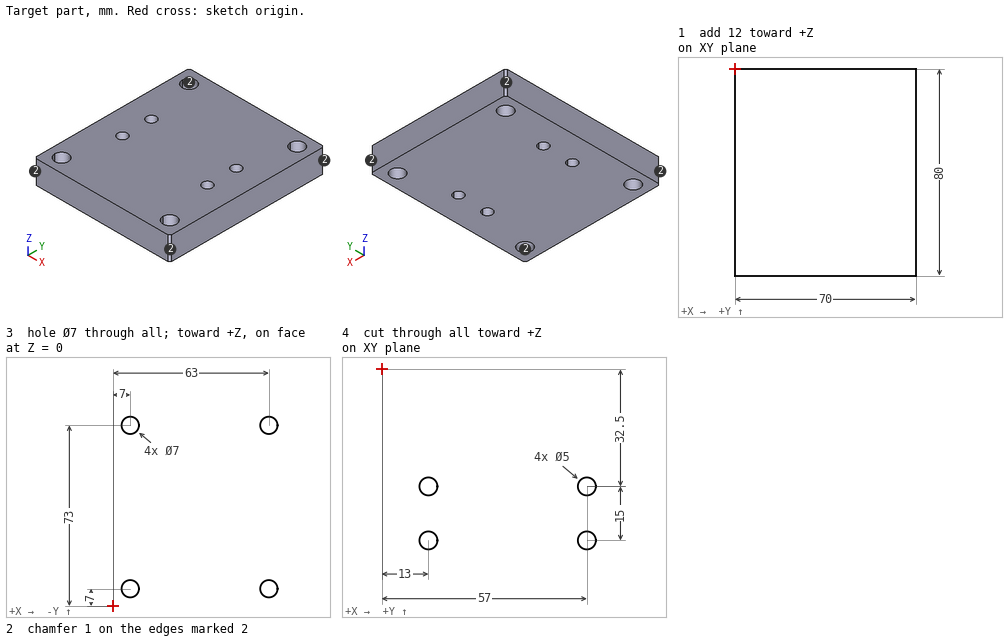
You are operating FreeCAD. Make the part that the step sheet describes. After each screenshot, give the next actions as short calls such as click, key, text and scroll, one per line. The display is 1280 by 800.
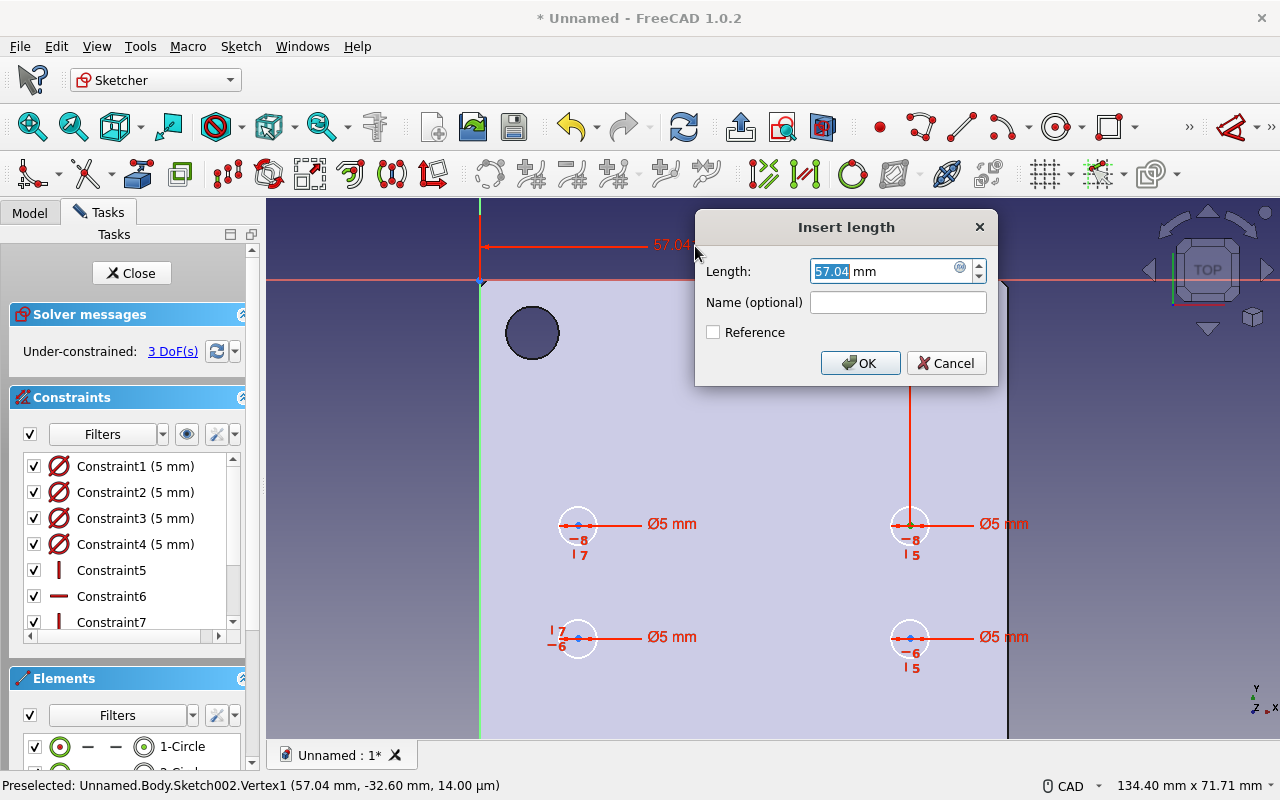
text(57)
key(Return)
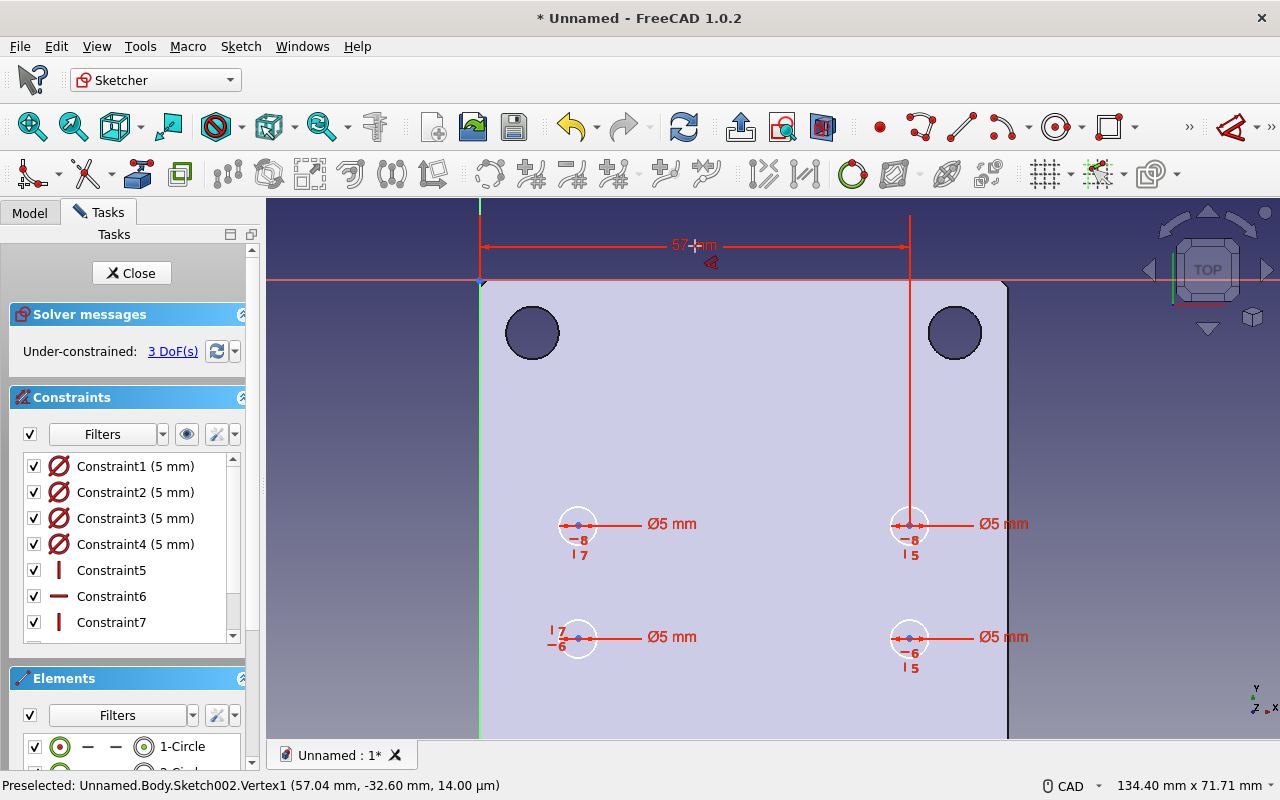
click(578, 639)
click(529, 246)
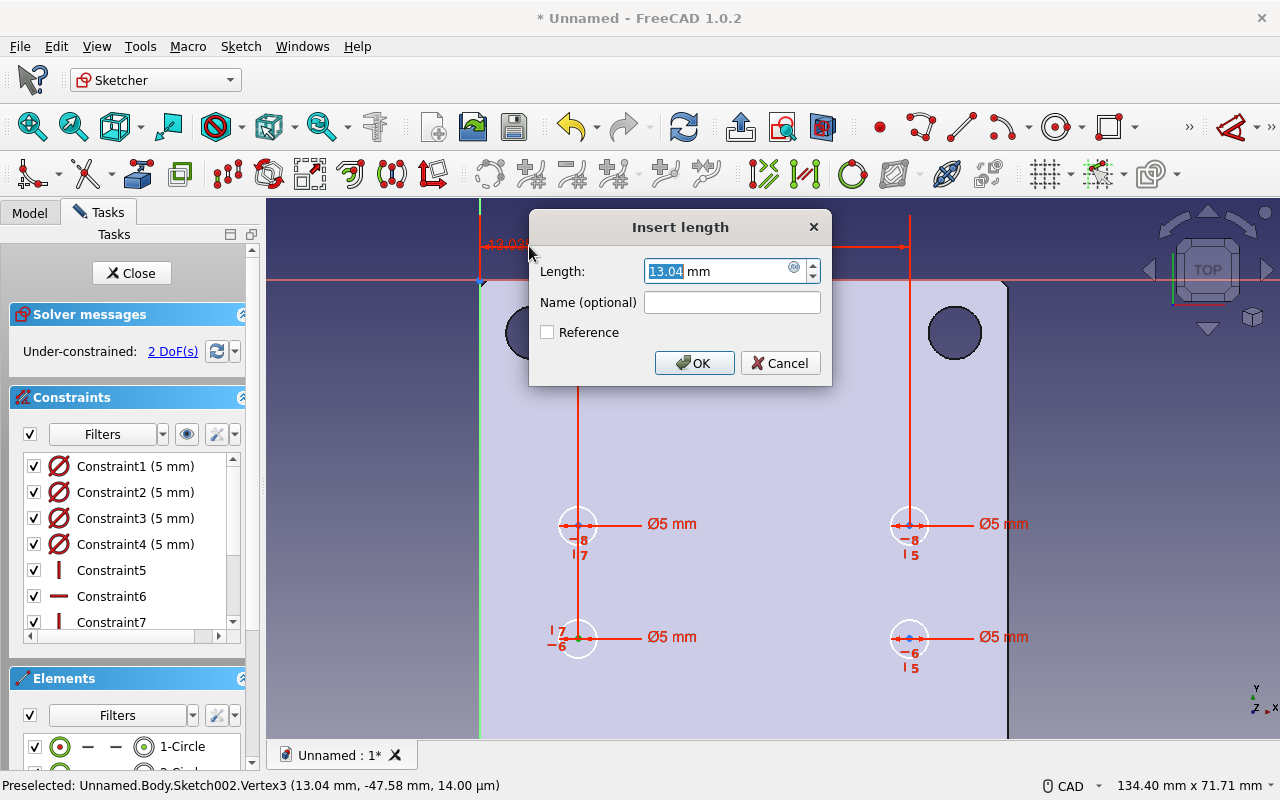
text(13)
key(Return)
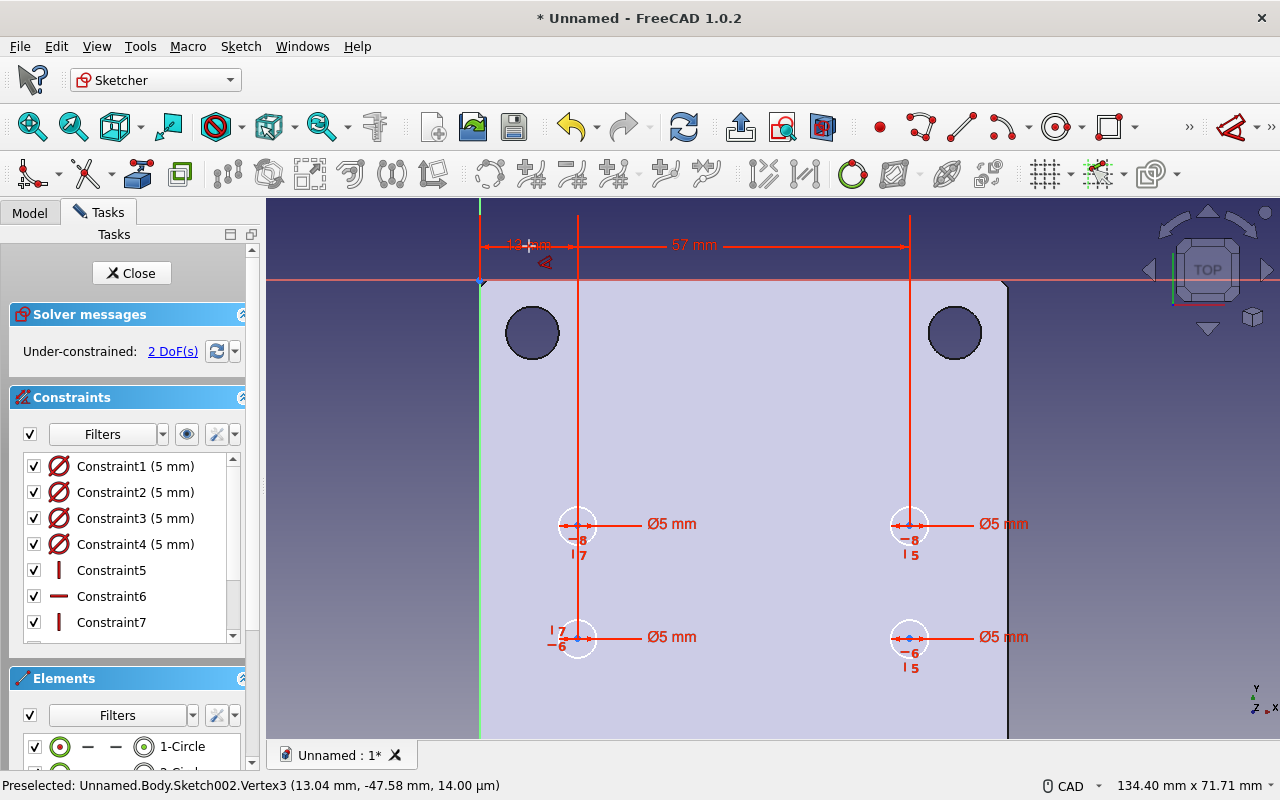
click(910, 526)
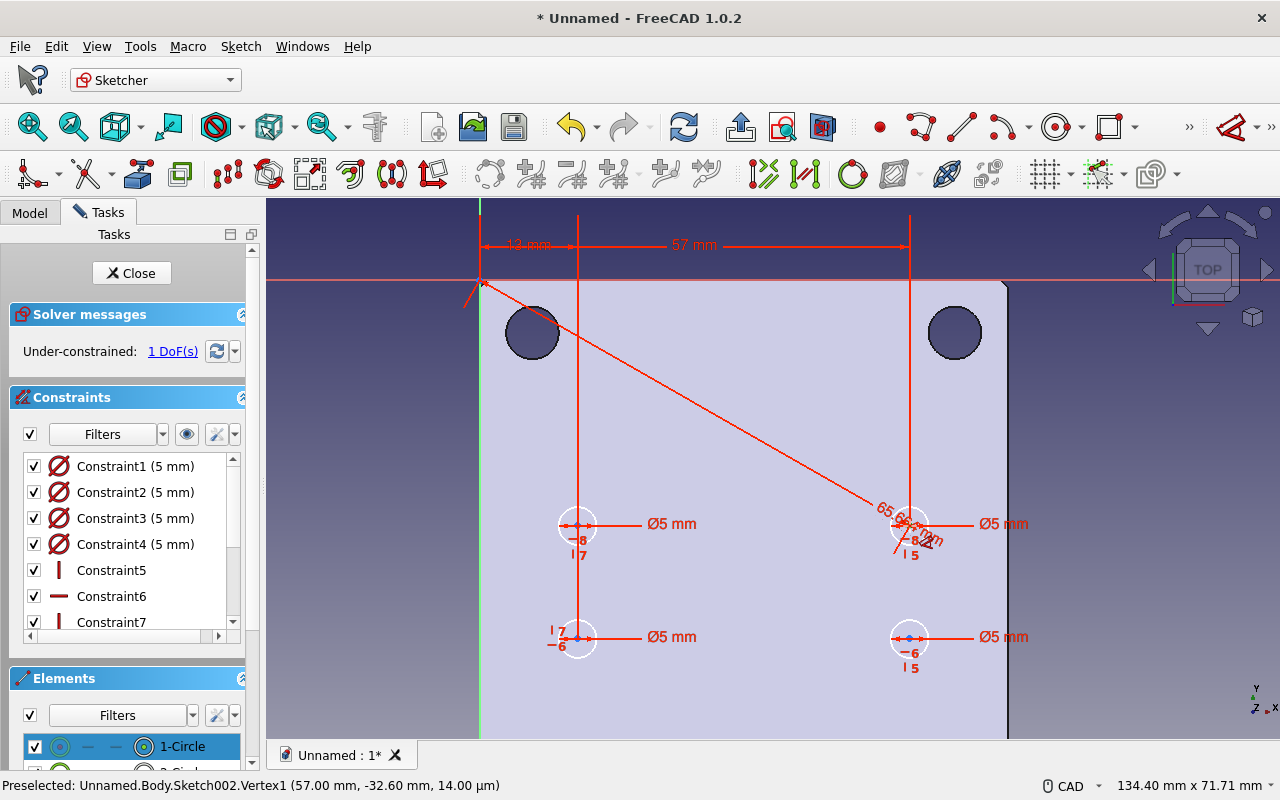
click(910, 639)
click(944, 582)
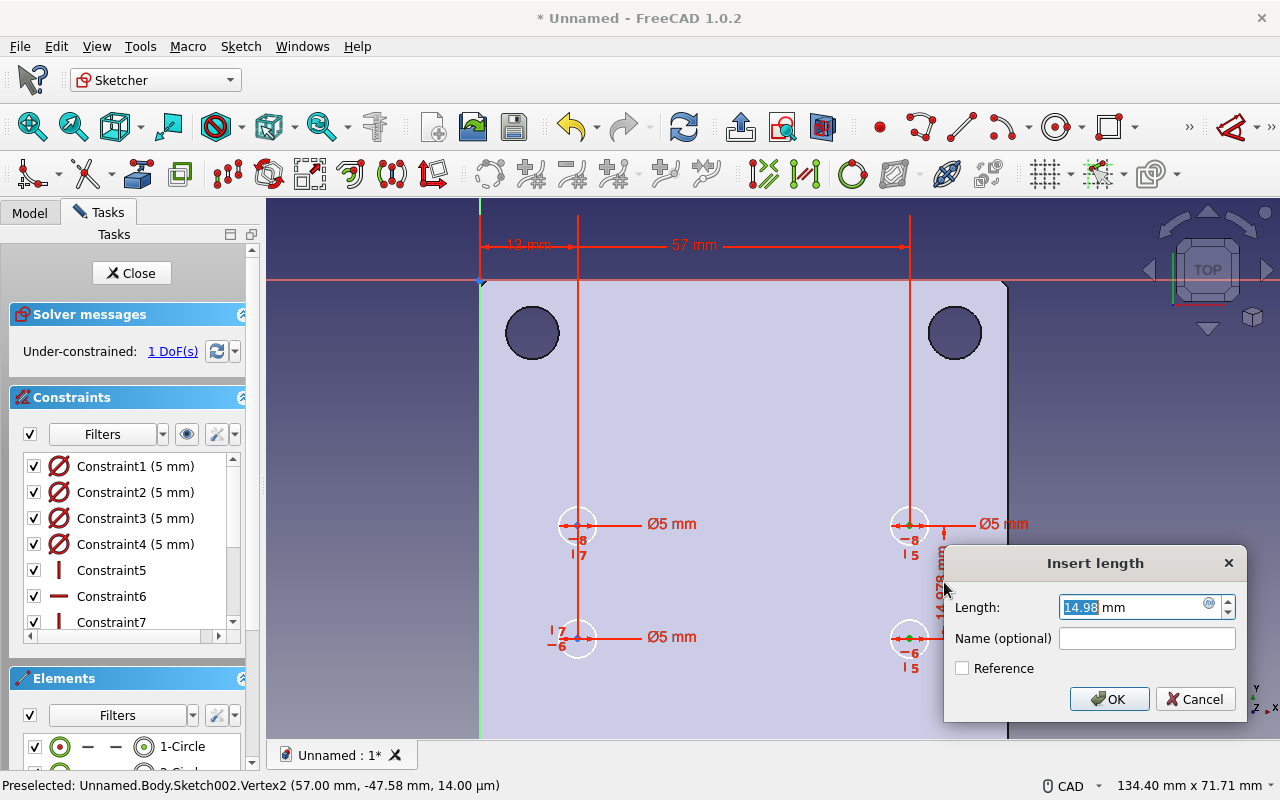
text(15)
key(Return)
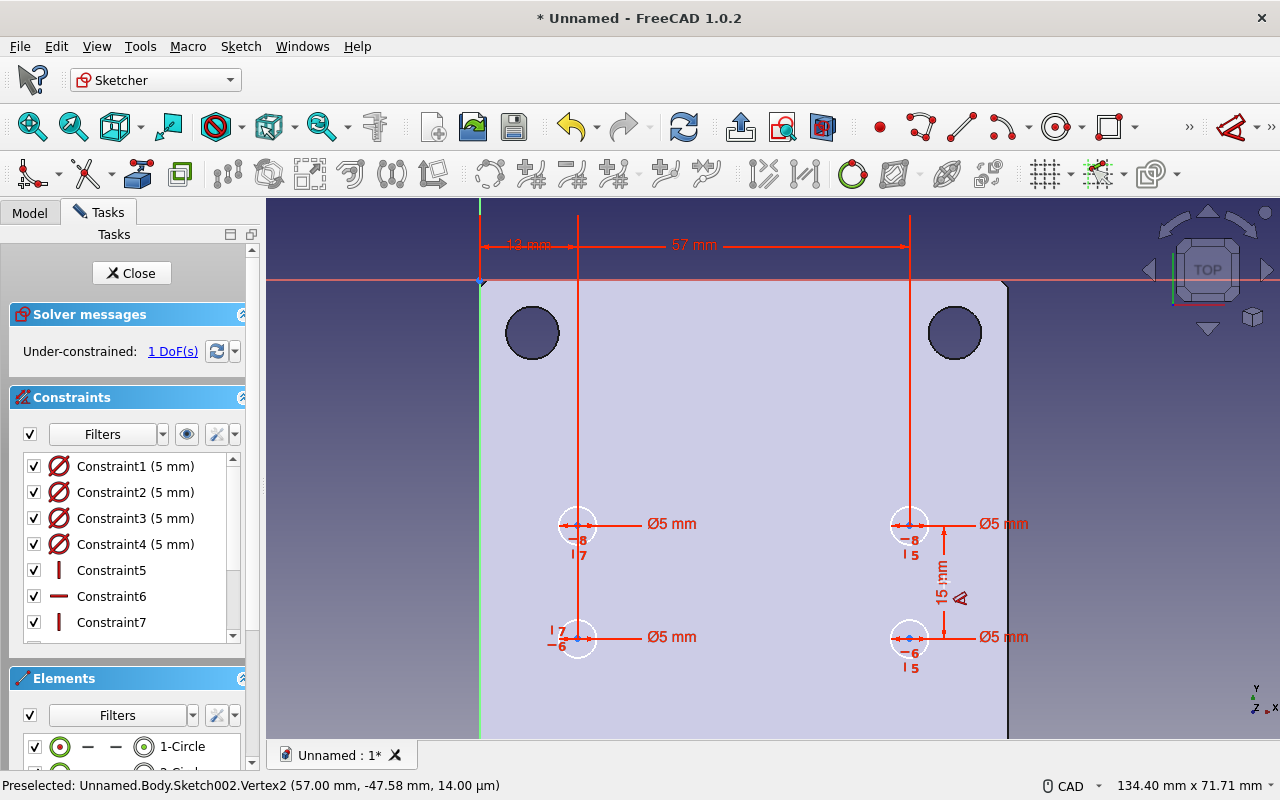
click(910, 526)
click(446, 403)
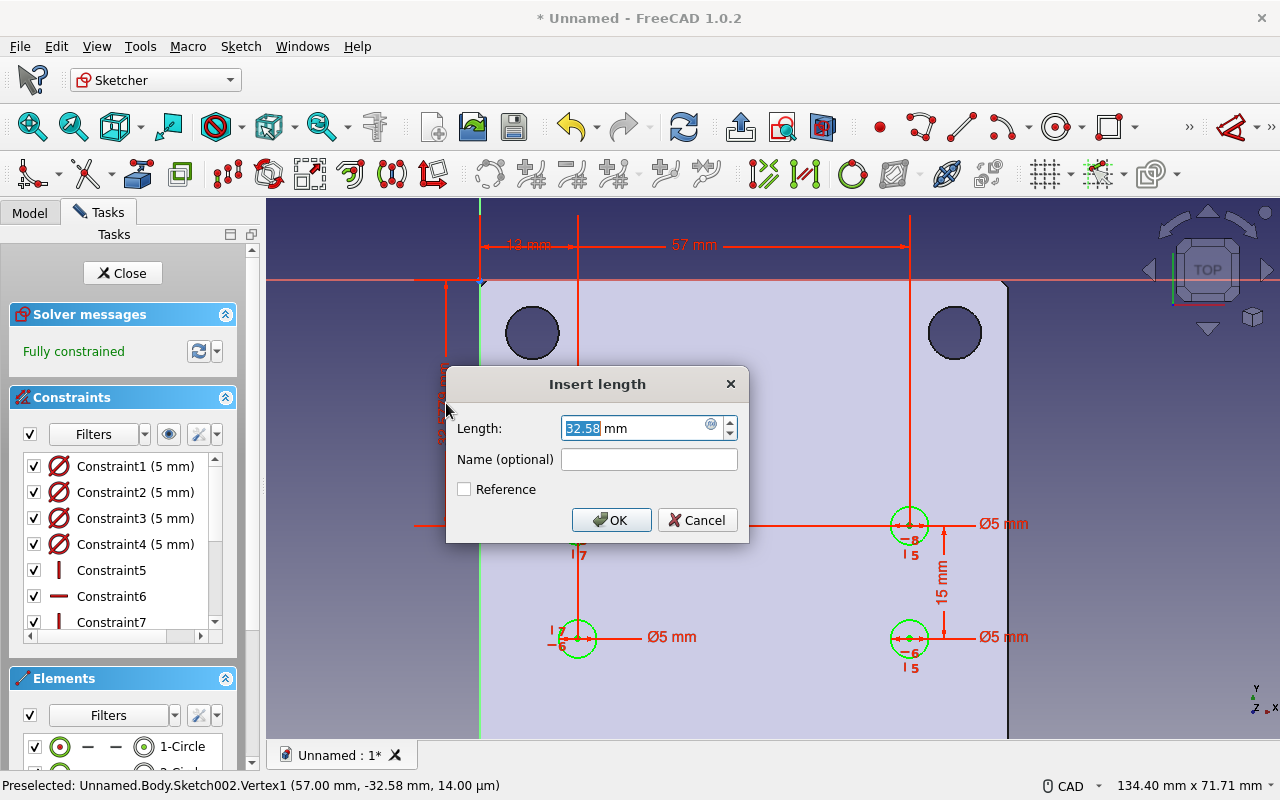
text(32.5)
key(Return)
key(Escape)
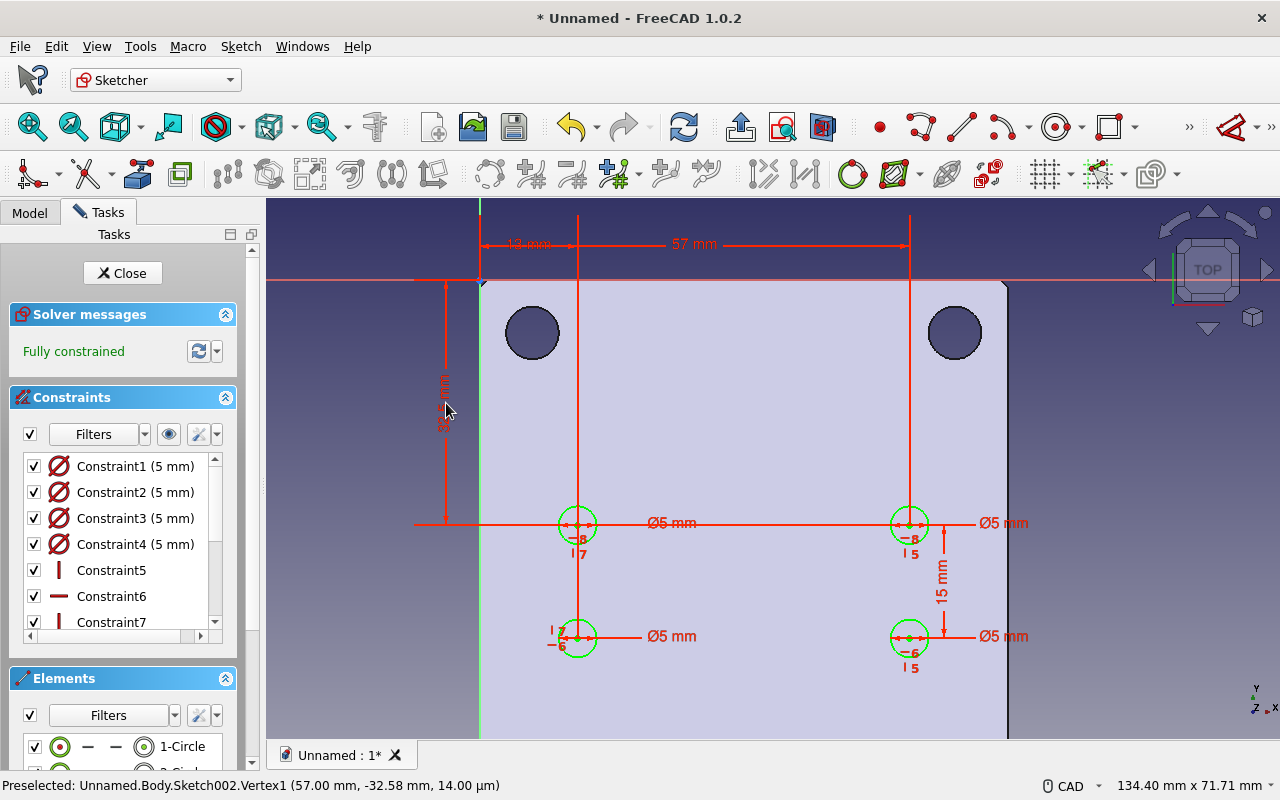
click(123, 273)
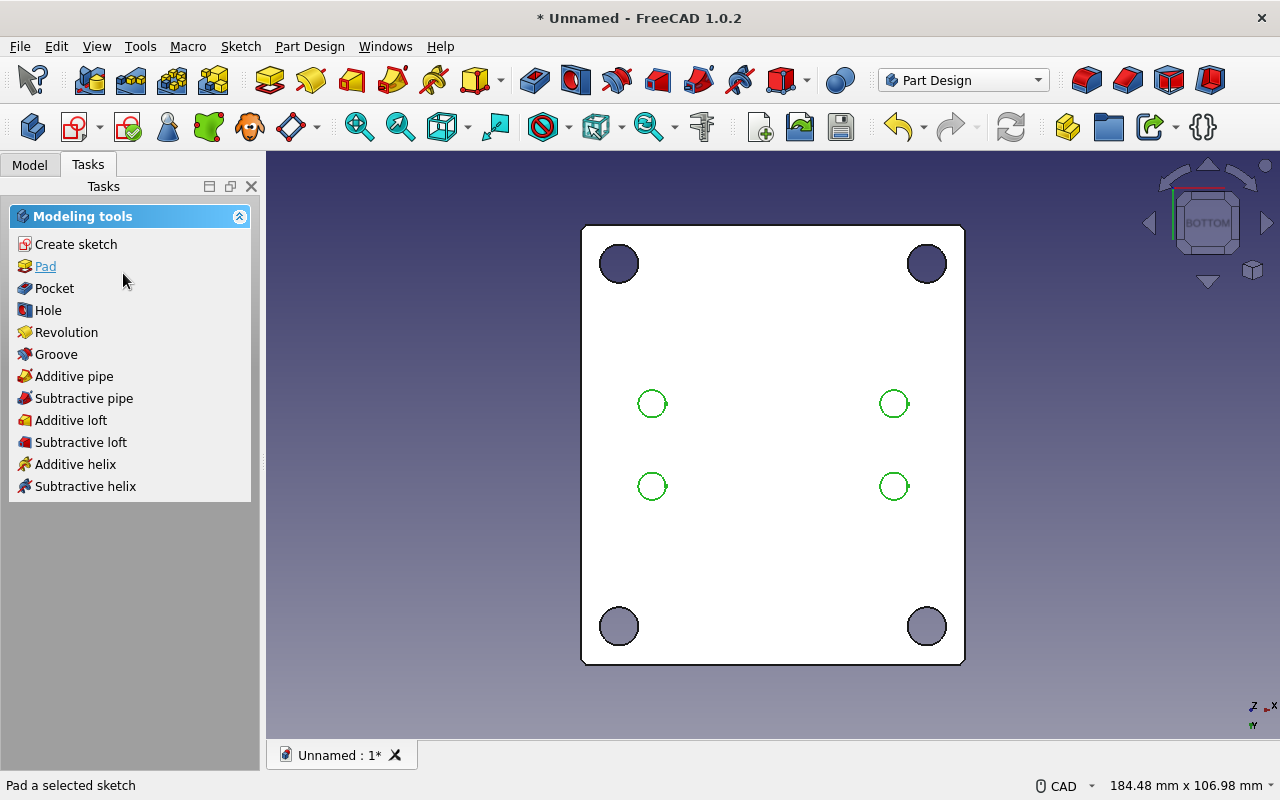
click(535, 80)